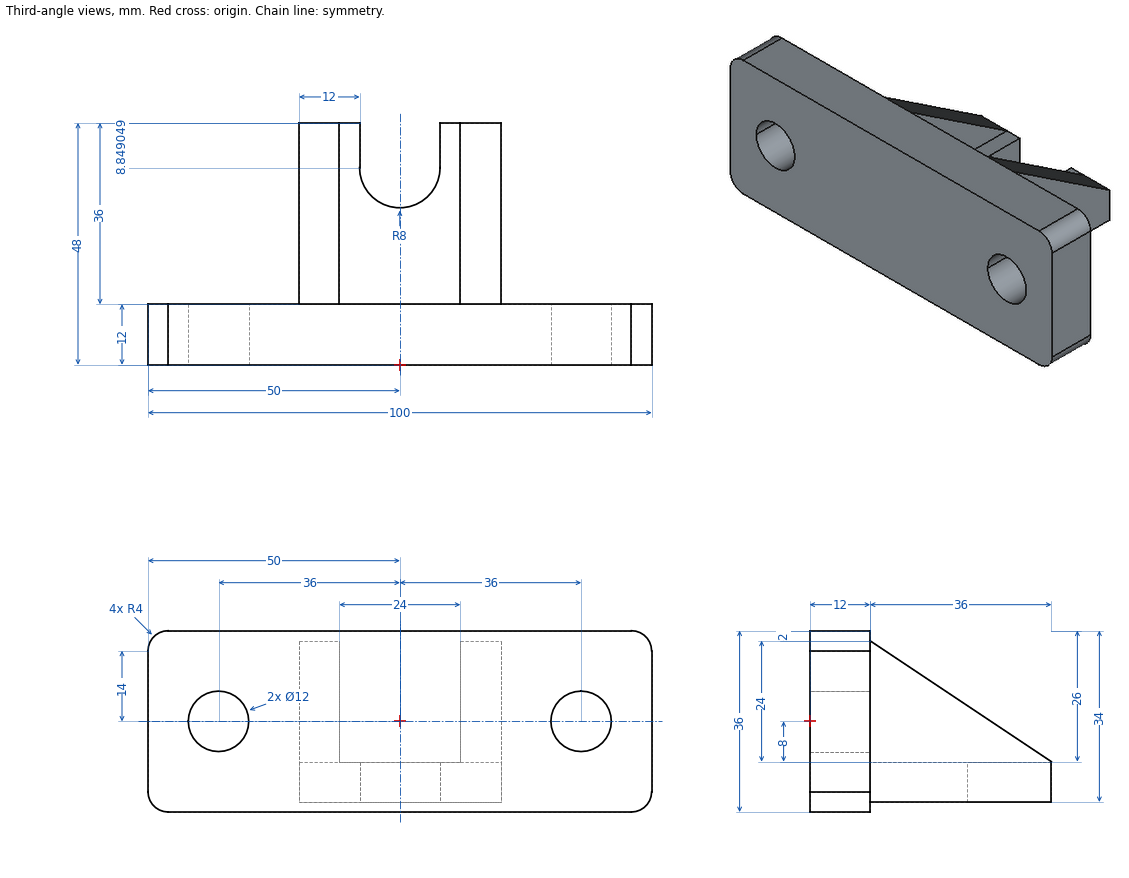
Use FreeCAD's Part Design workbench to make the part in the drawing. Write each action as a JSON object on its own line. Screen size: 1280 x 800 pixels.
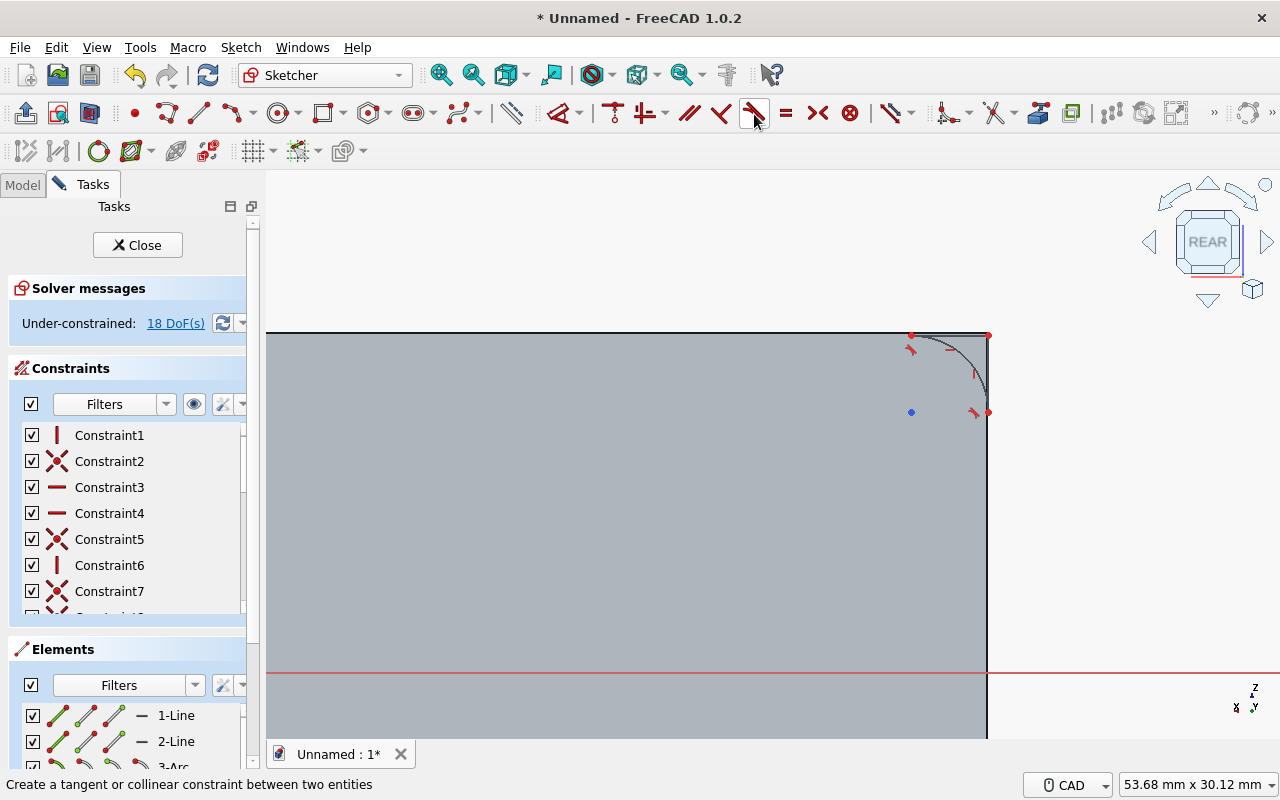
{"action": "scroll", "coordinate": [990, 360], "scroll_direction": "down", "scroll_amount": 6}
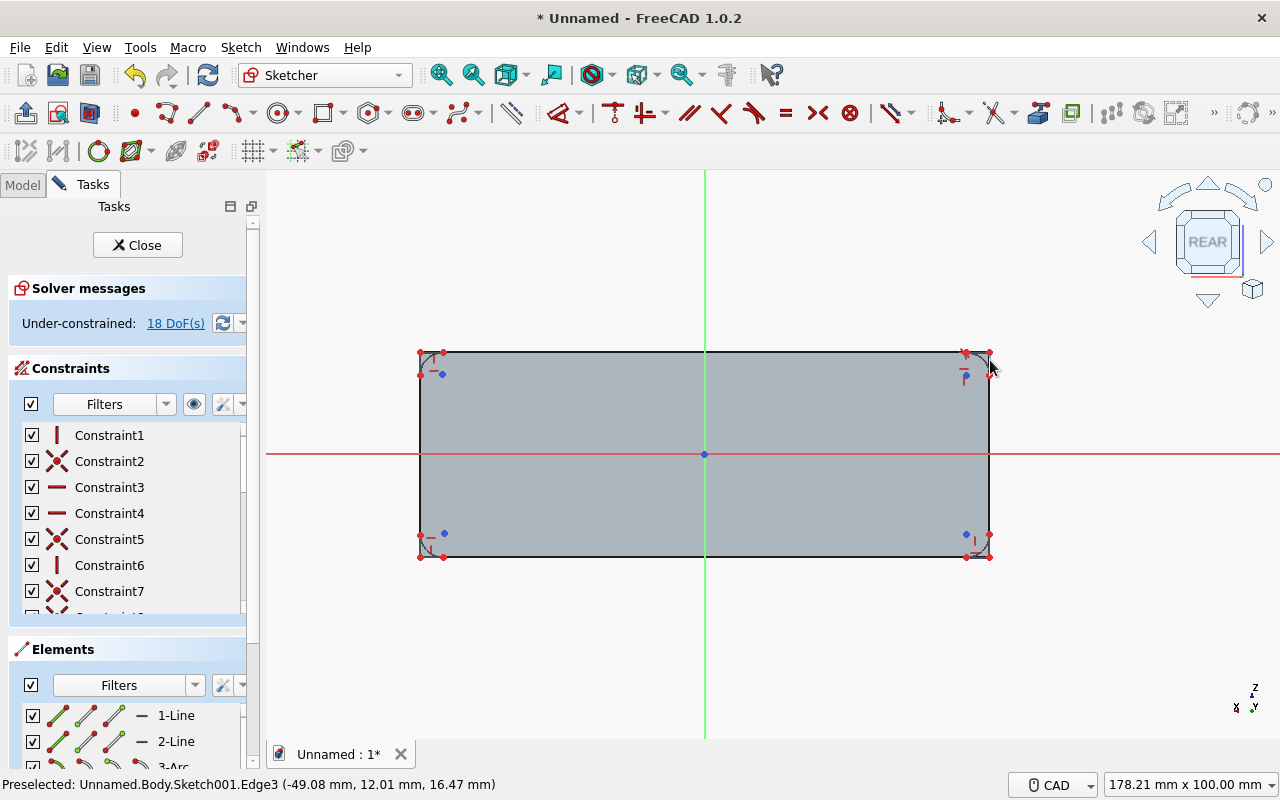
{"action": "scroll", "coordinate": [427, 353], "scroll_direction": "up", "scroll_amount": 6}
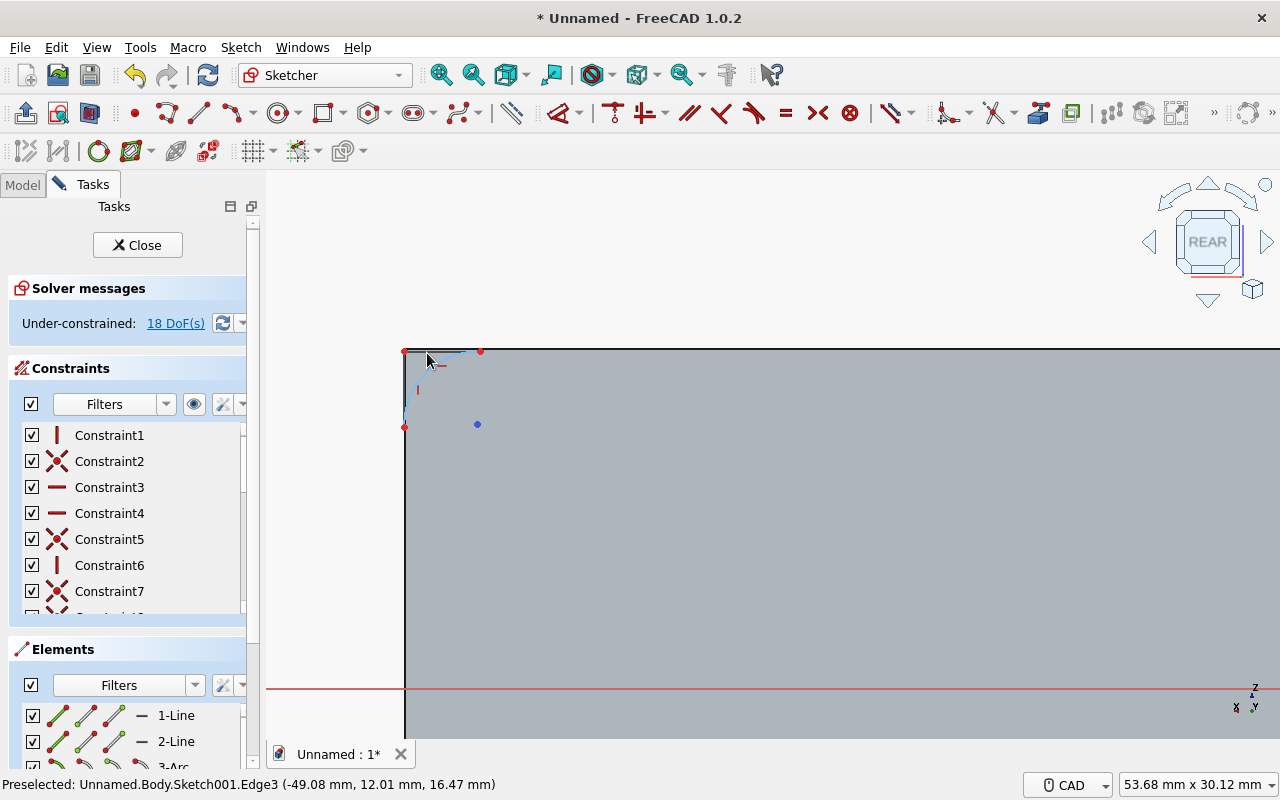
{"action": "left_click", "coordinate": [427, 352]}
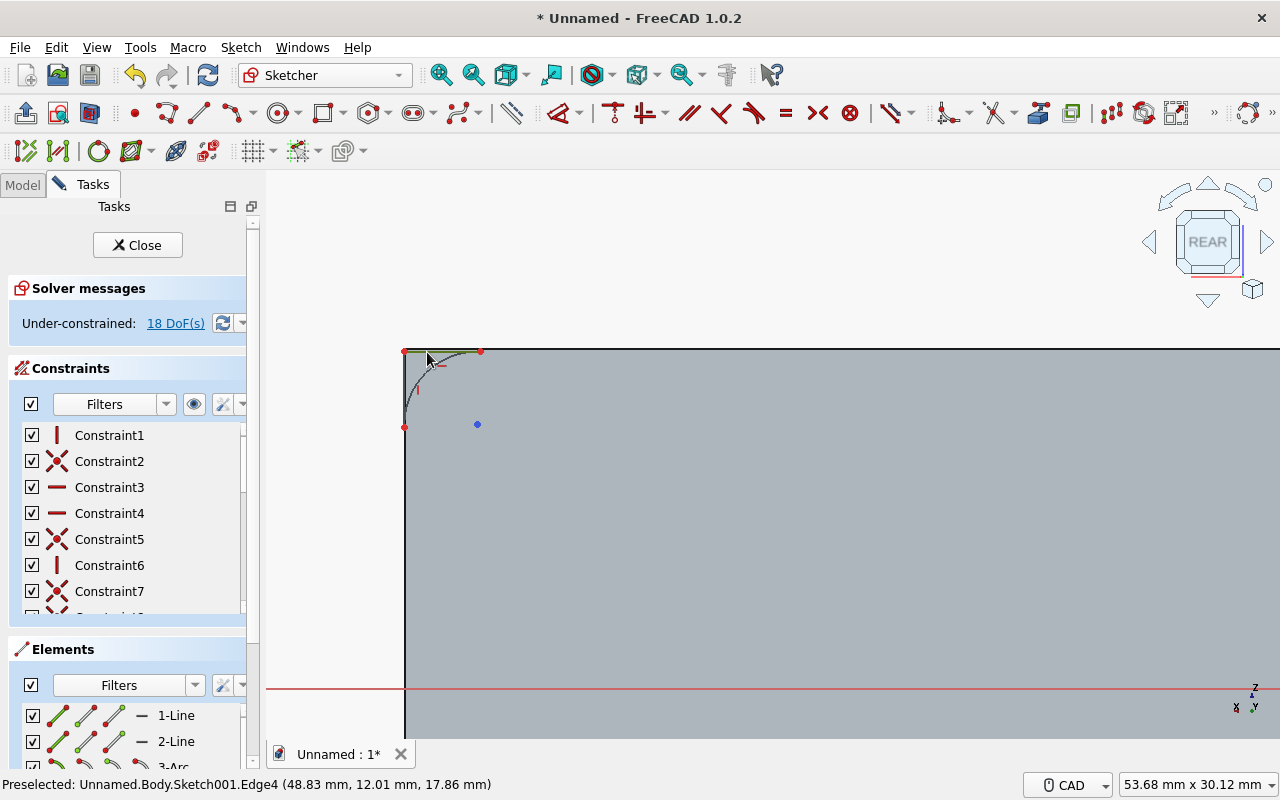
{"action": "left_click", "coordinate": [426, 373]}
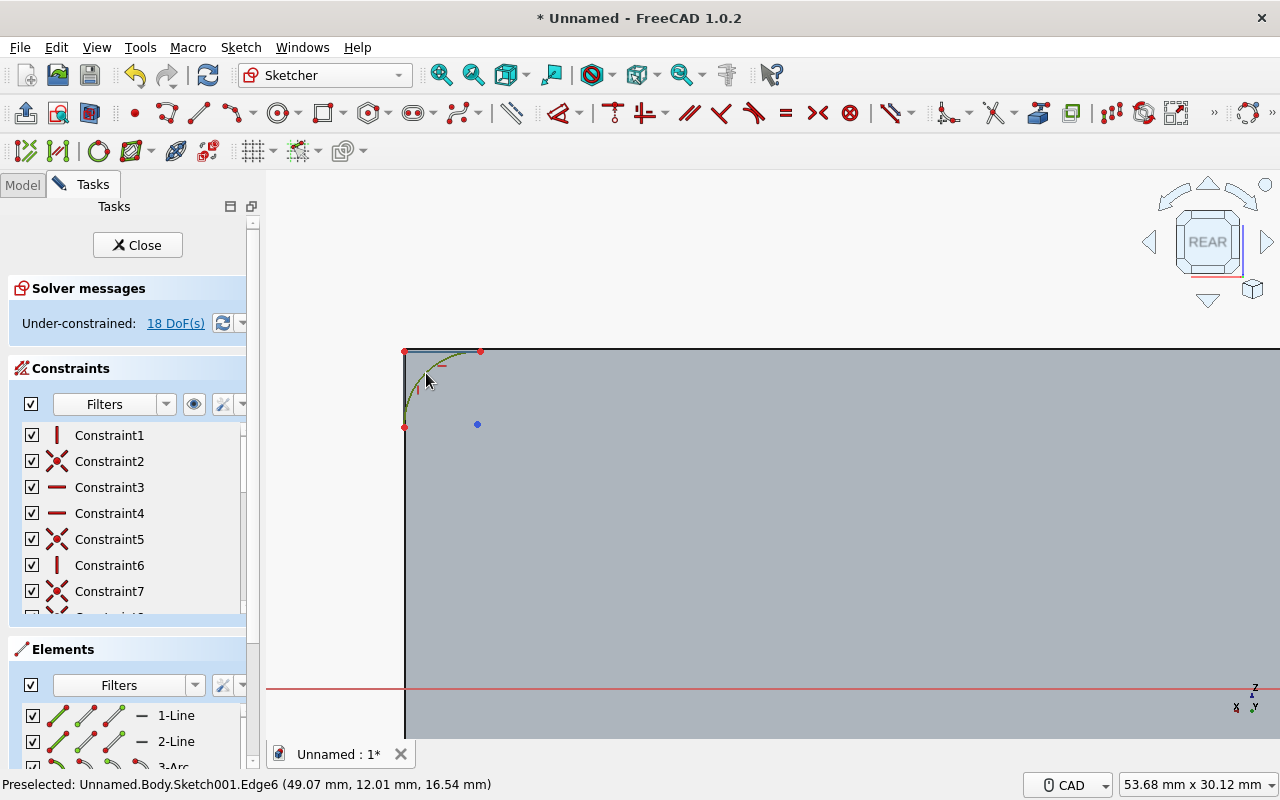
{"action": "left_click", "coordinate": [754, 114]}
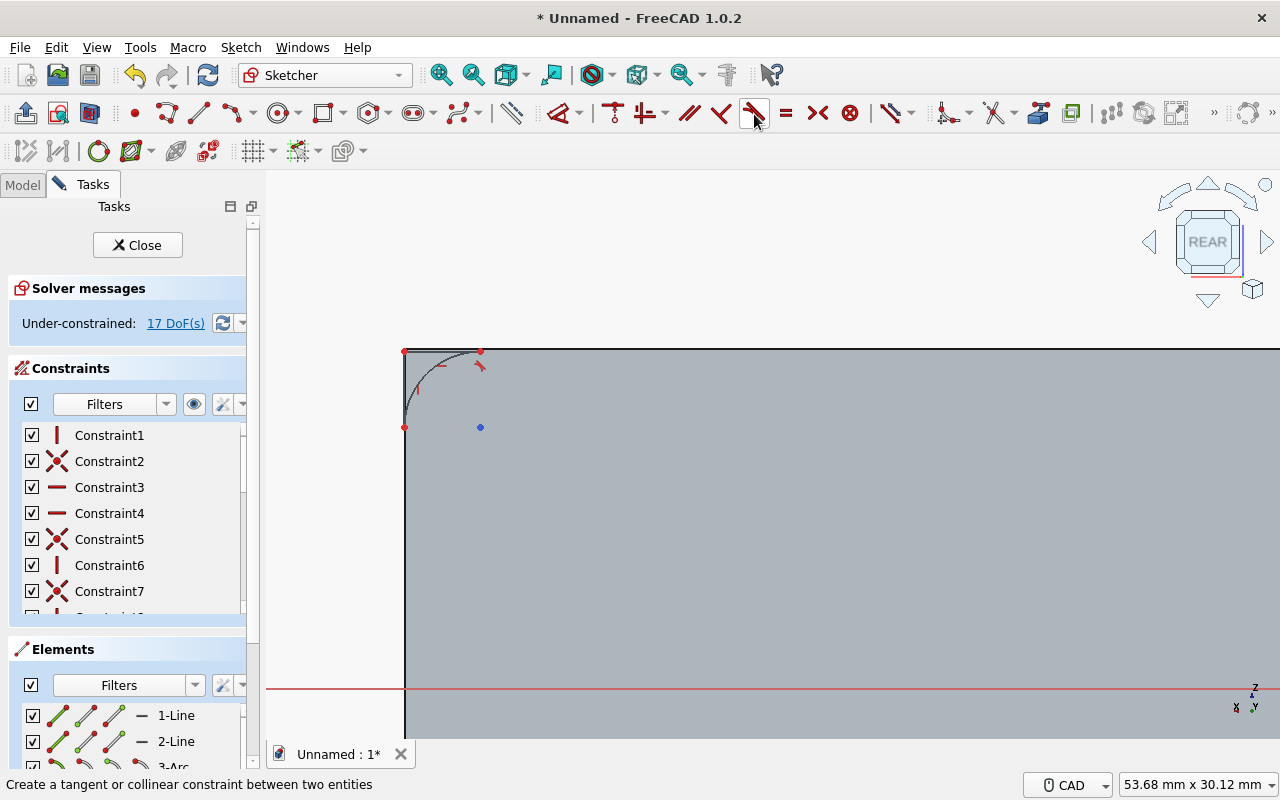
{"action": "left_click", "coordinate": [404, 374]}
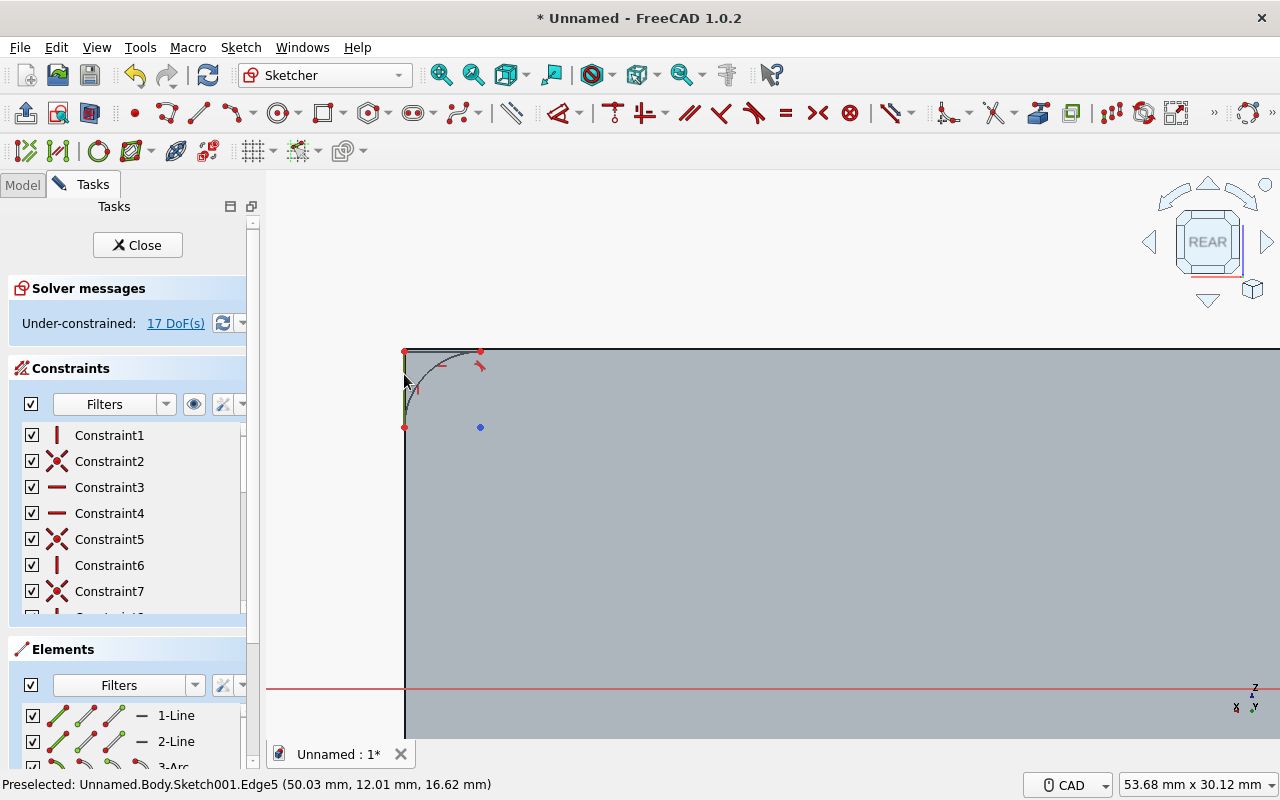
{"action": "left_click", "coordinate": [427, 374]}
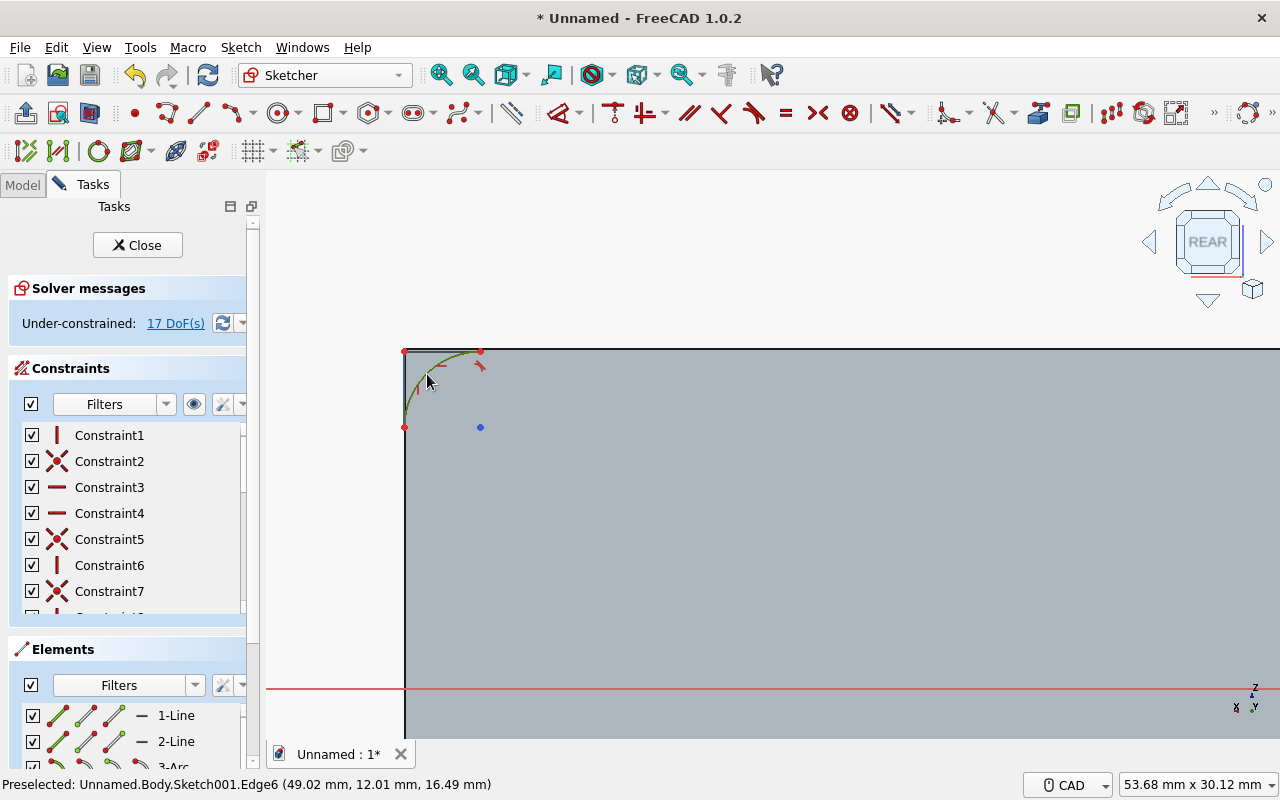
{"action": "left_click", "coordinate": [754, 114]}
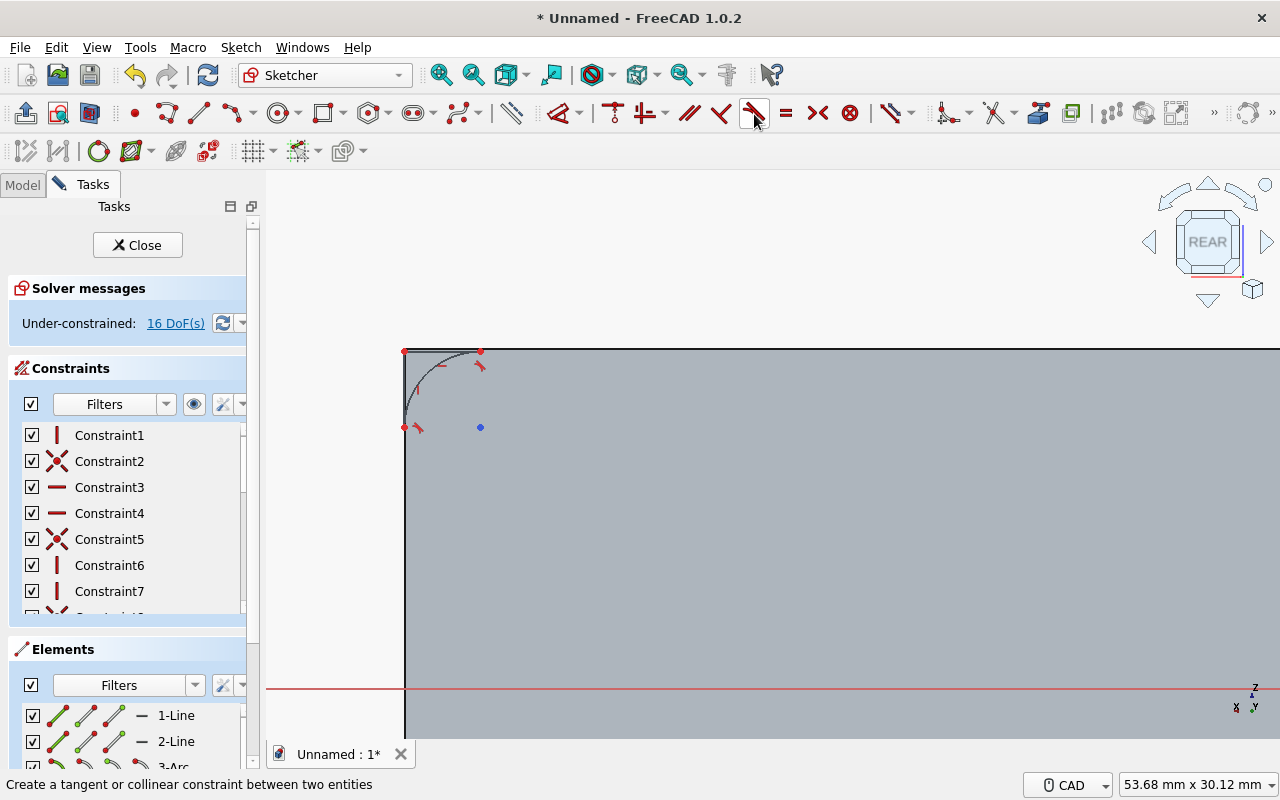
{"action": "scroll", "coordinate": [426, 353], "scroll_direction": "down", "scroll_amount": 6}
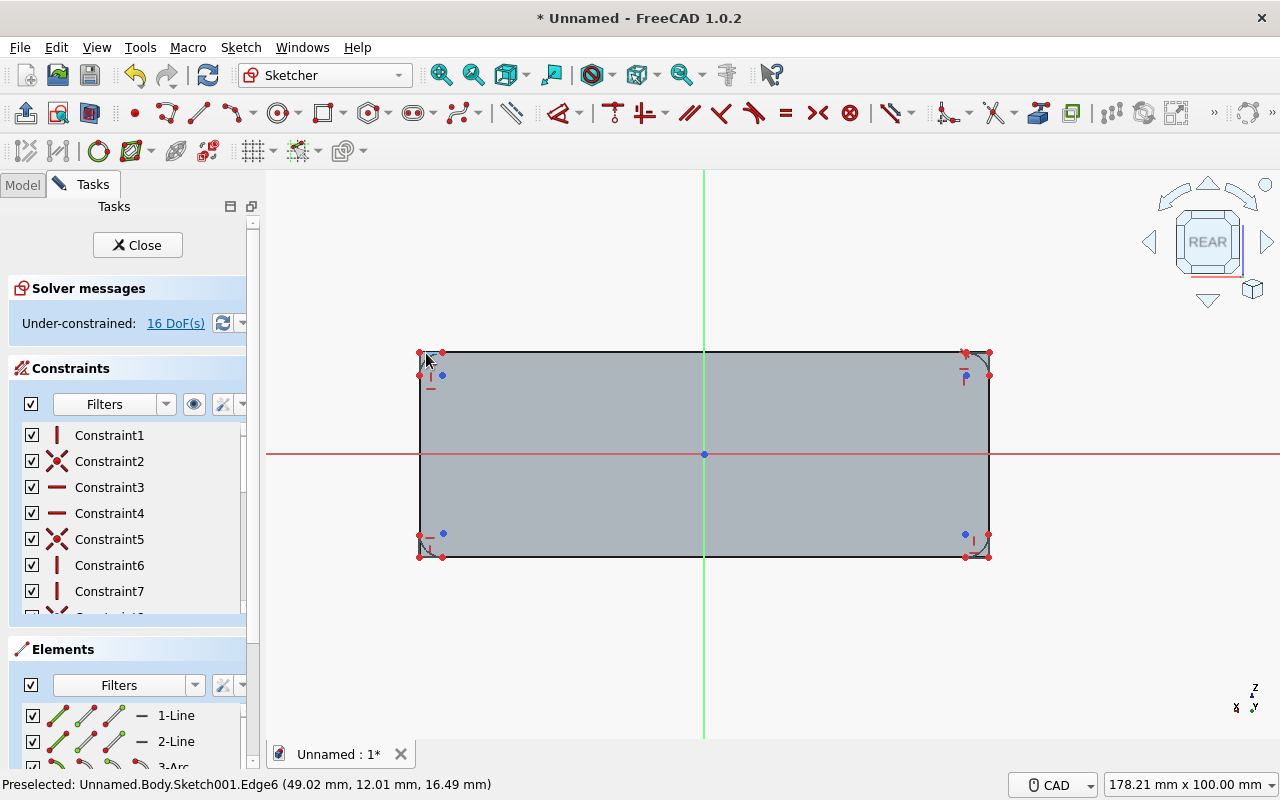
{"action": "scroll", "coordinate": [419, 551], "scroll_direction": "up", "scroll_amount": 5}